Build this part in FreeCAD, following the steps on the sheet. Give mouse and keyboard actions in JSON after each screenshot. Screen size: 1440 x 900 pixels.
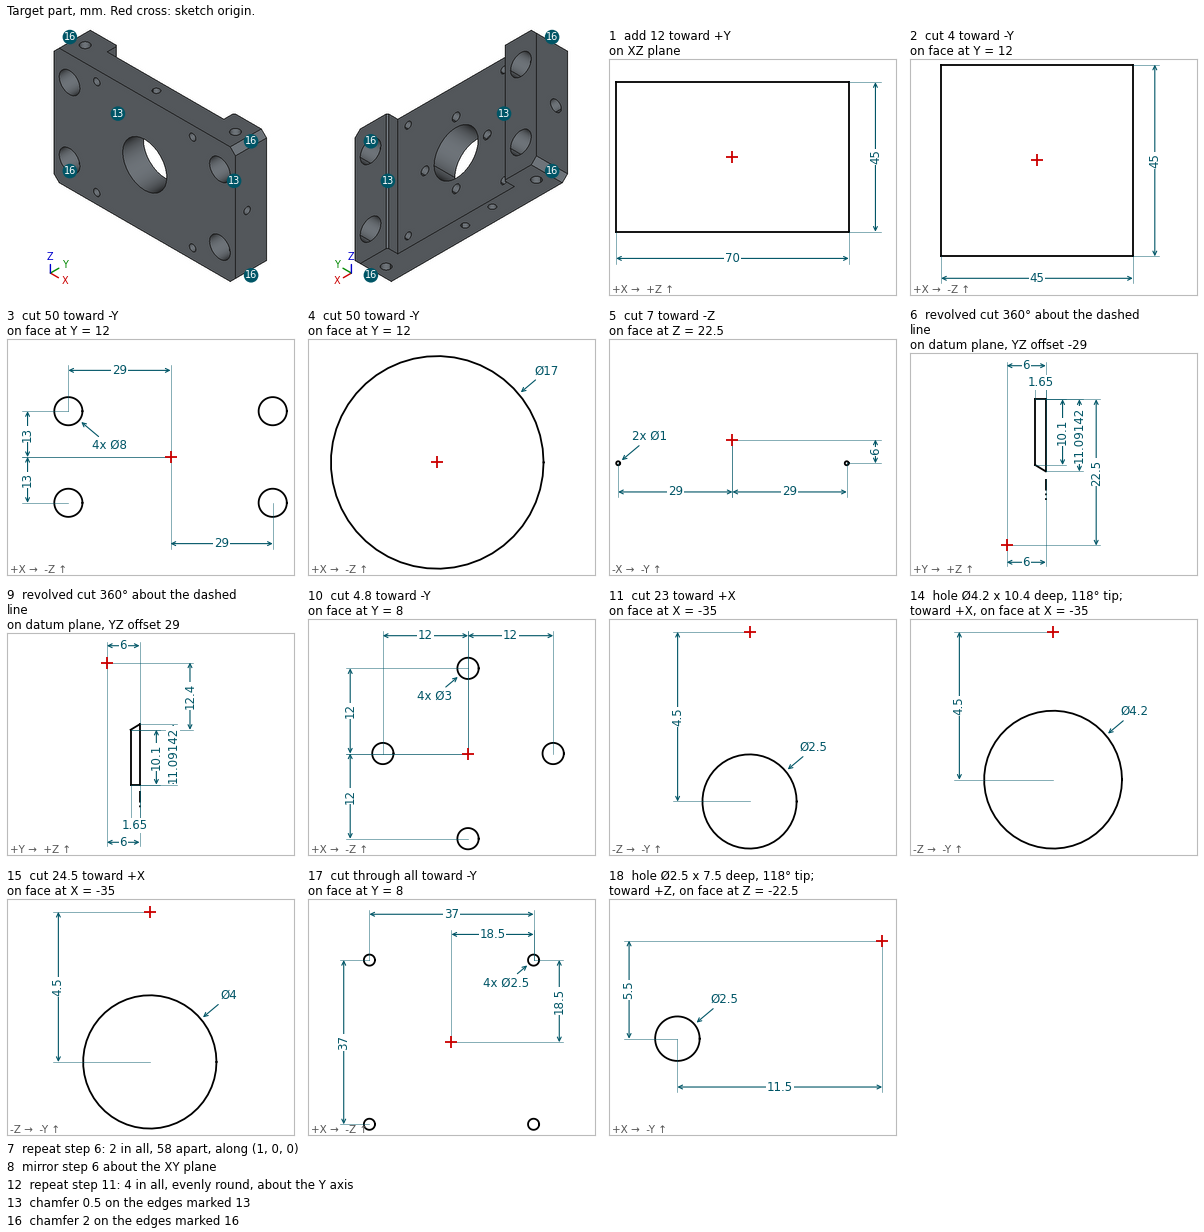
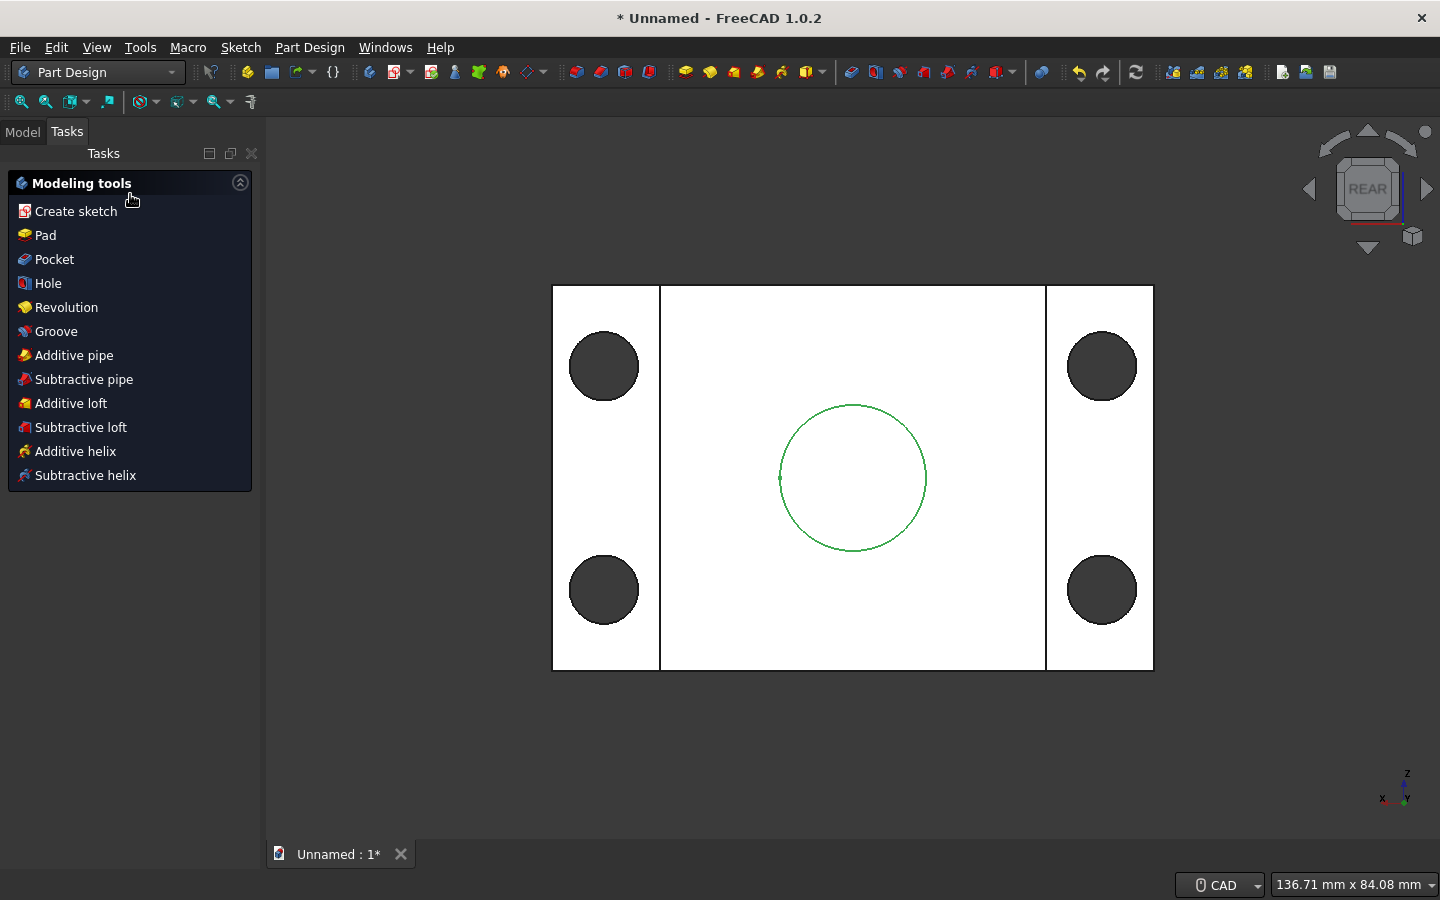
{"action": "left_click", "coordinate": [852, 72]}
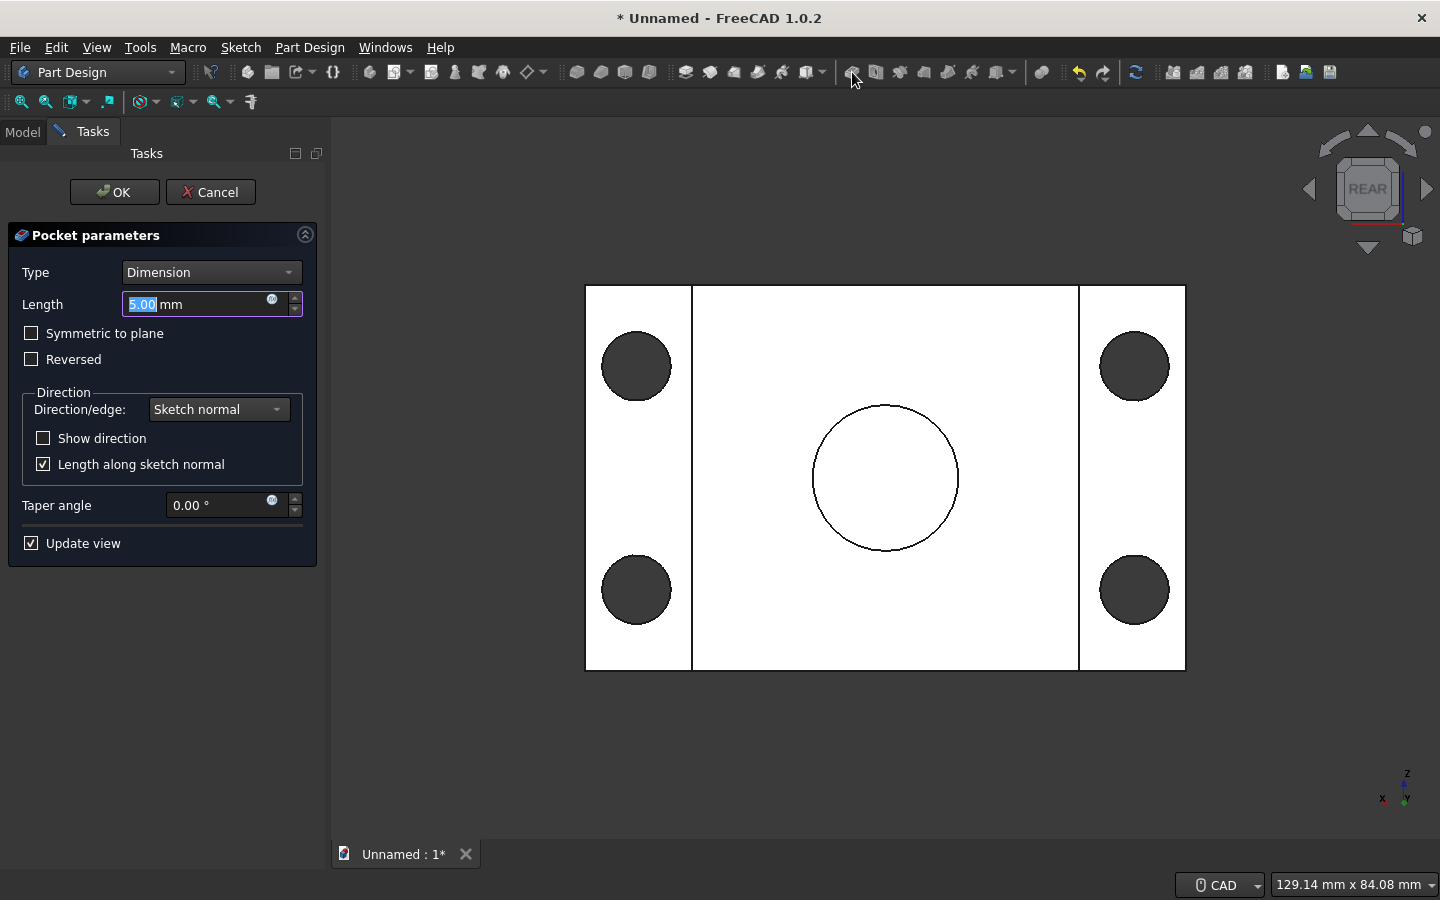
{"action": "type", "text": "50"}
{"action": "key", "text": "Tab"}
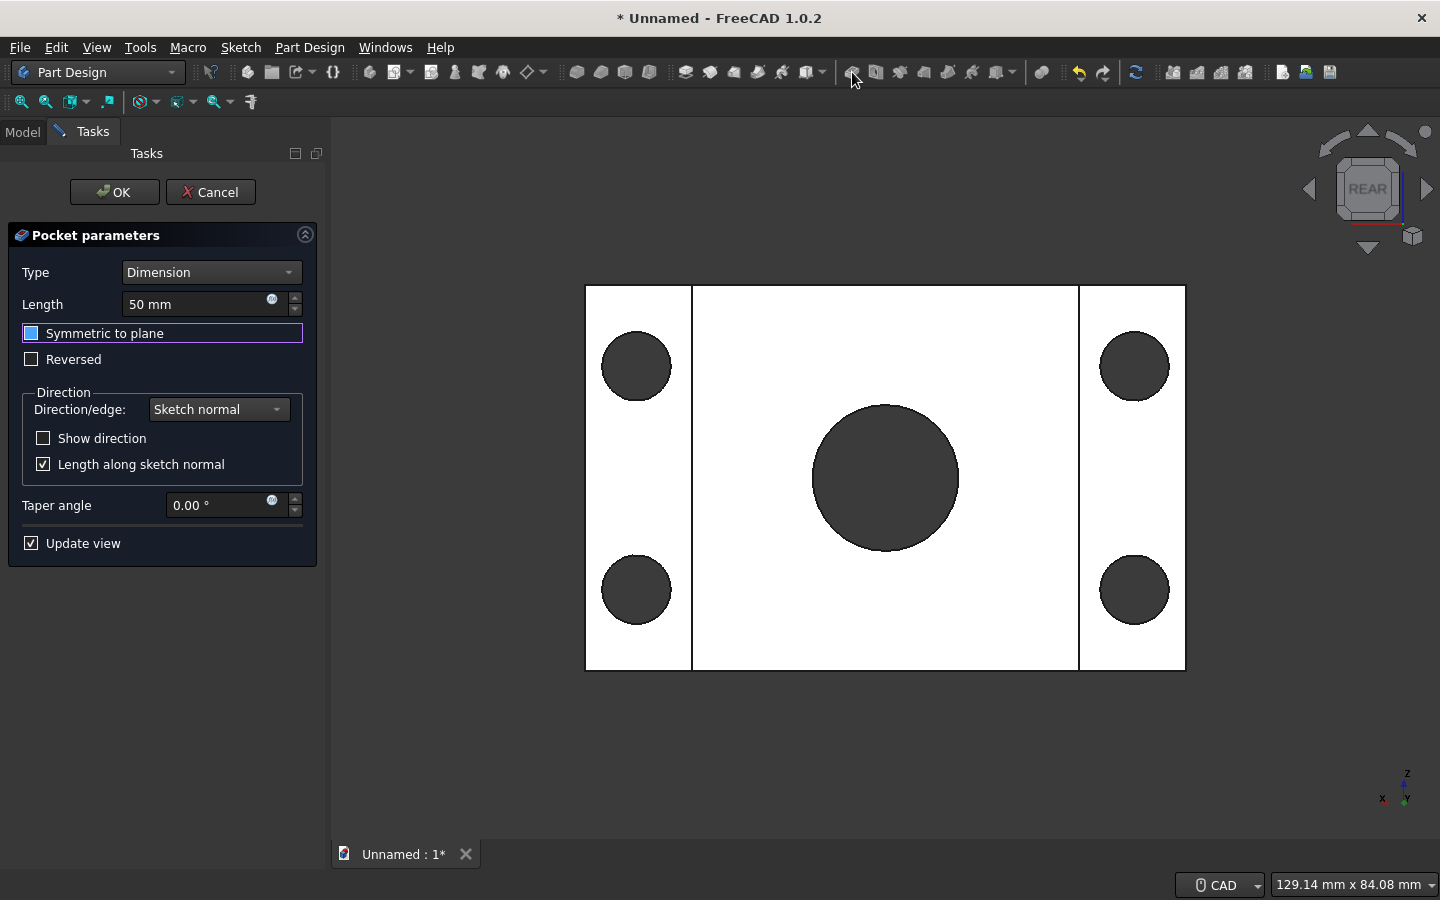
{"action": "left_click", "coordinate": [115, 192]}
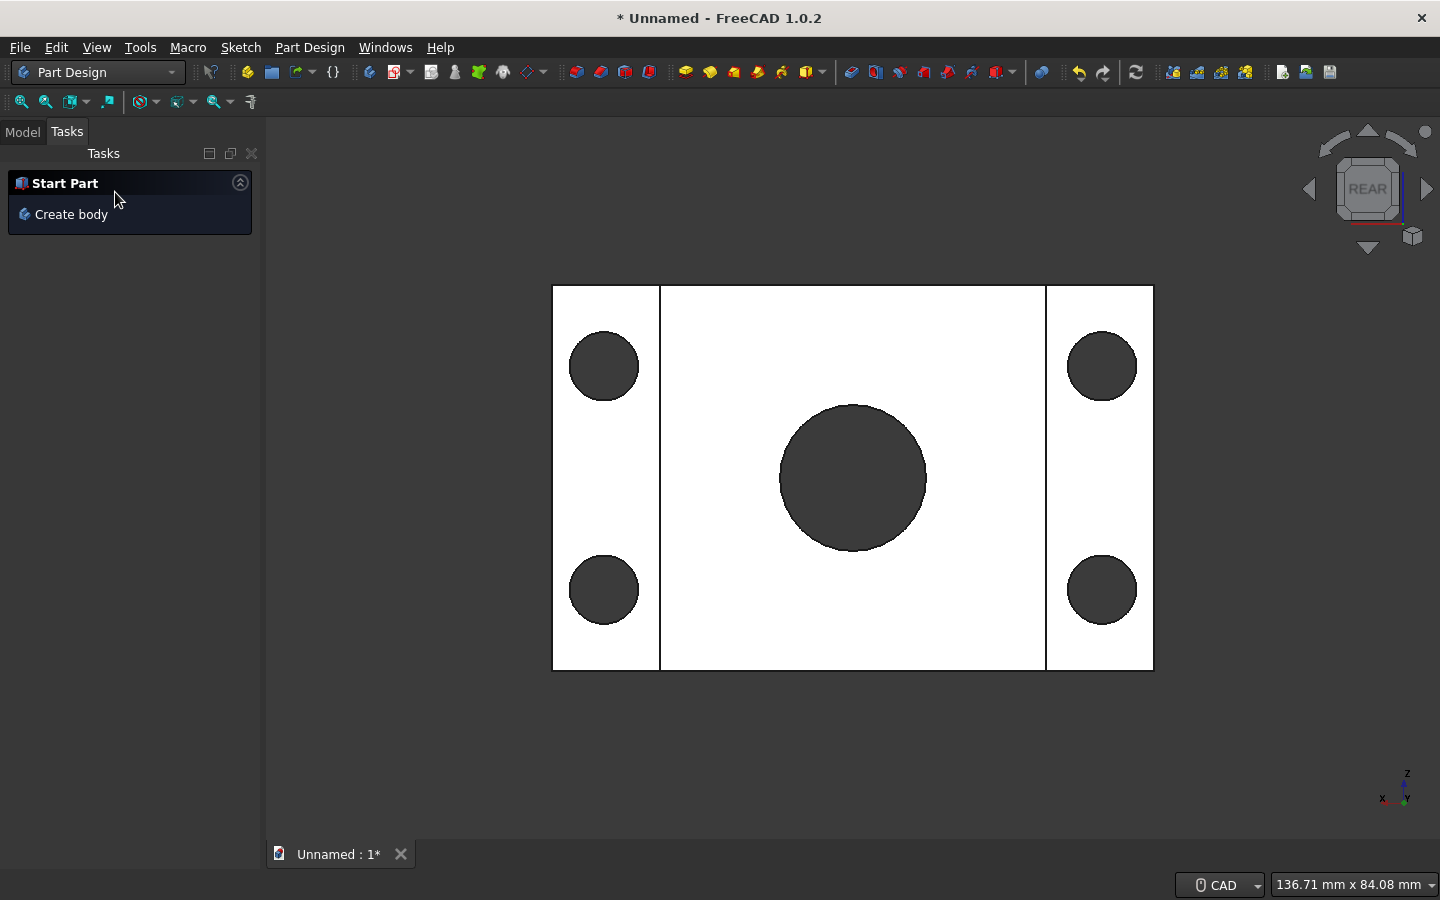
{"action": "key", "text": "0"}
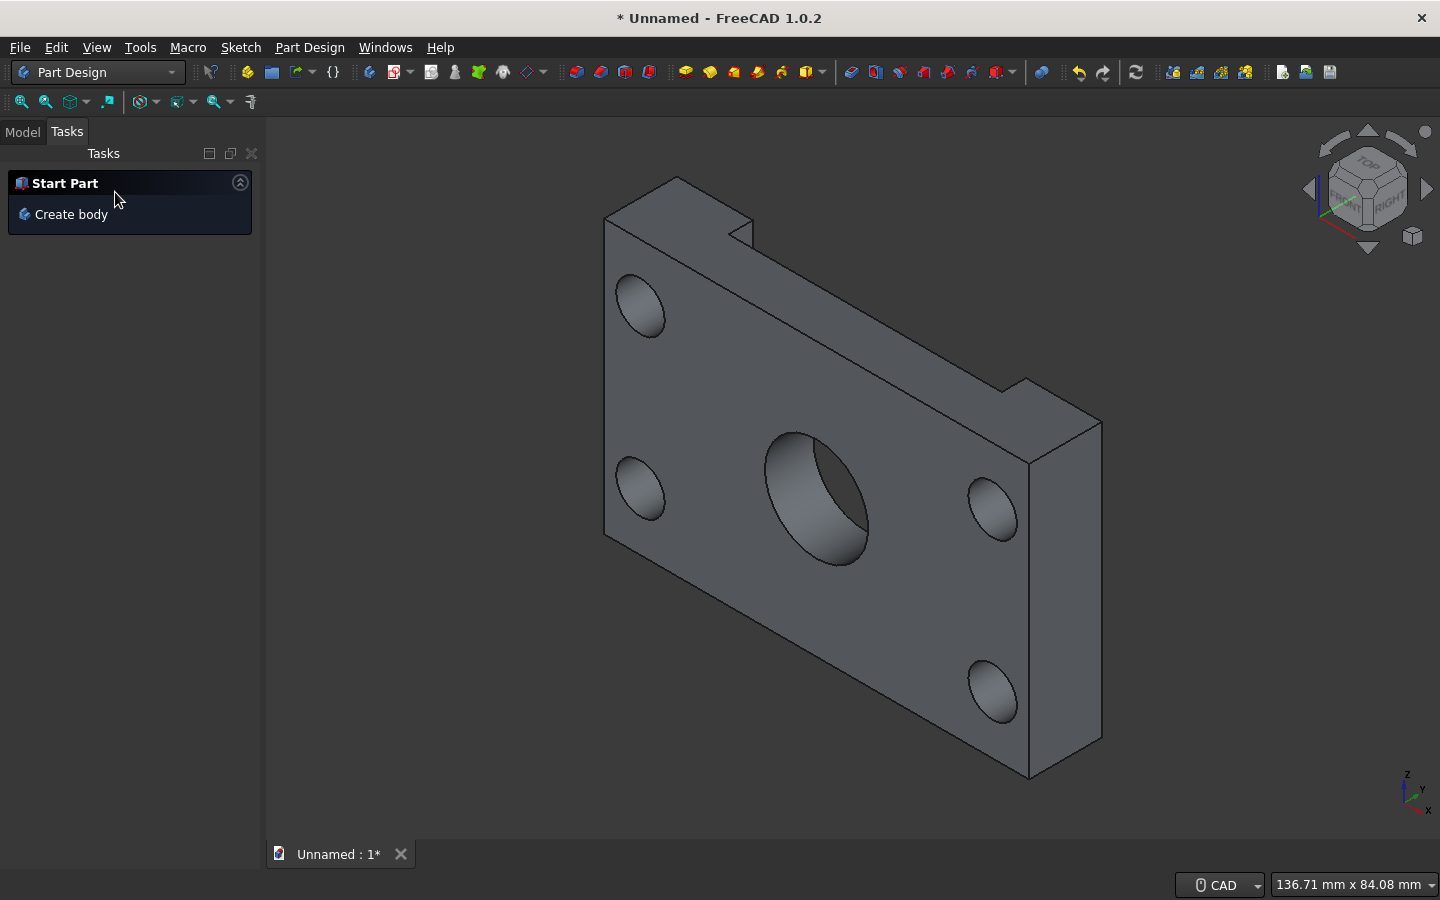
{"action": "left_click", "coordinate": [1035, 424]}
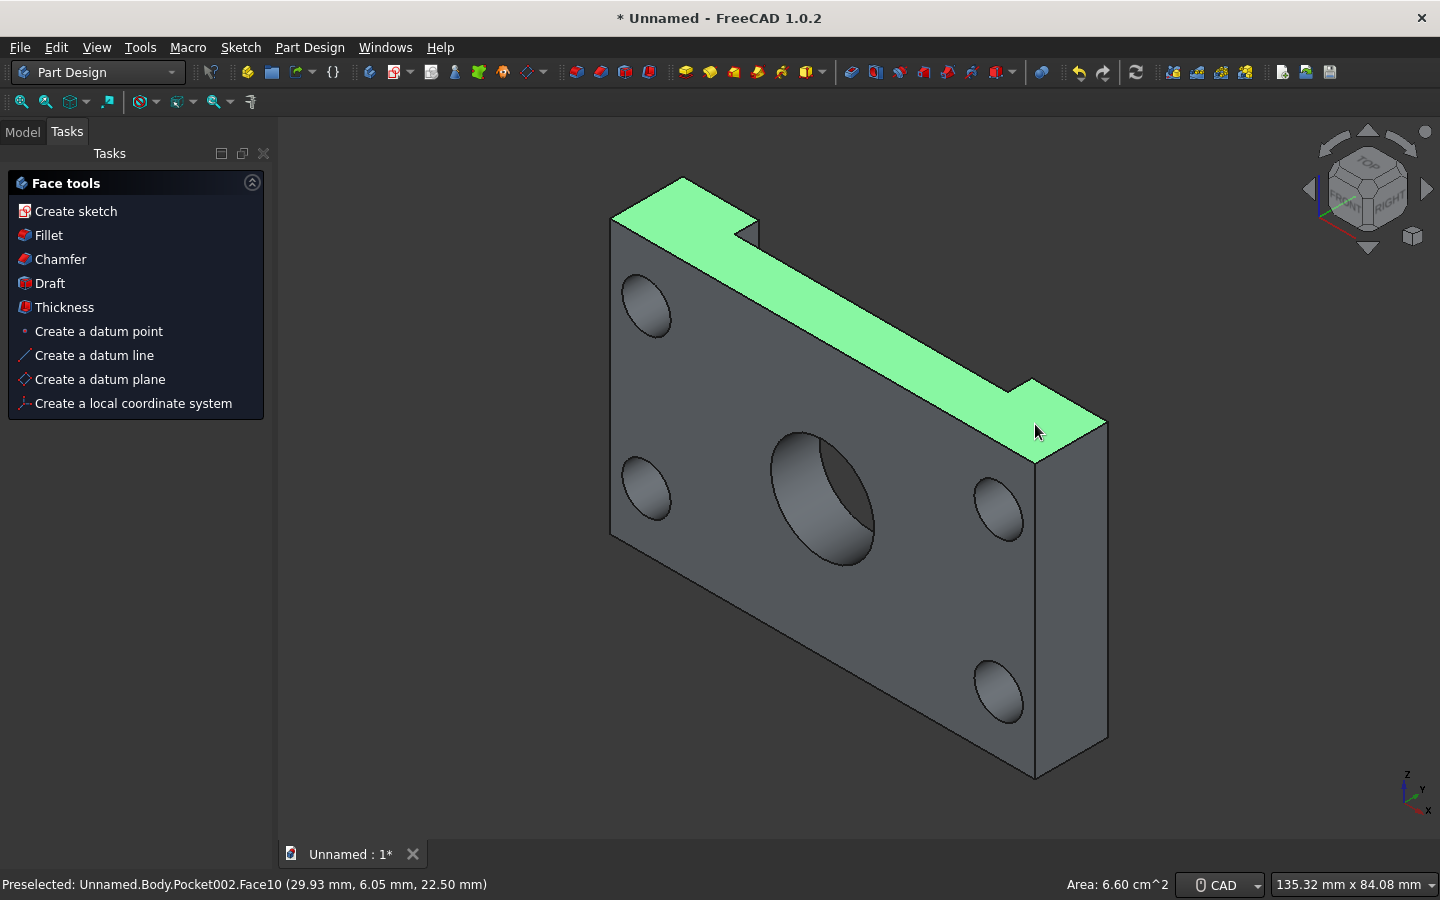
{"action": "left_click", "coordinate": [394, 72]}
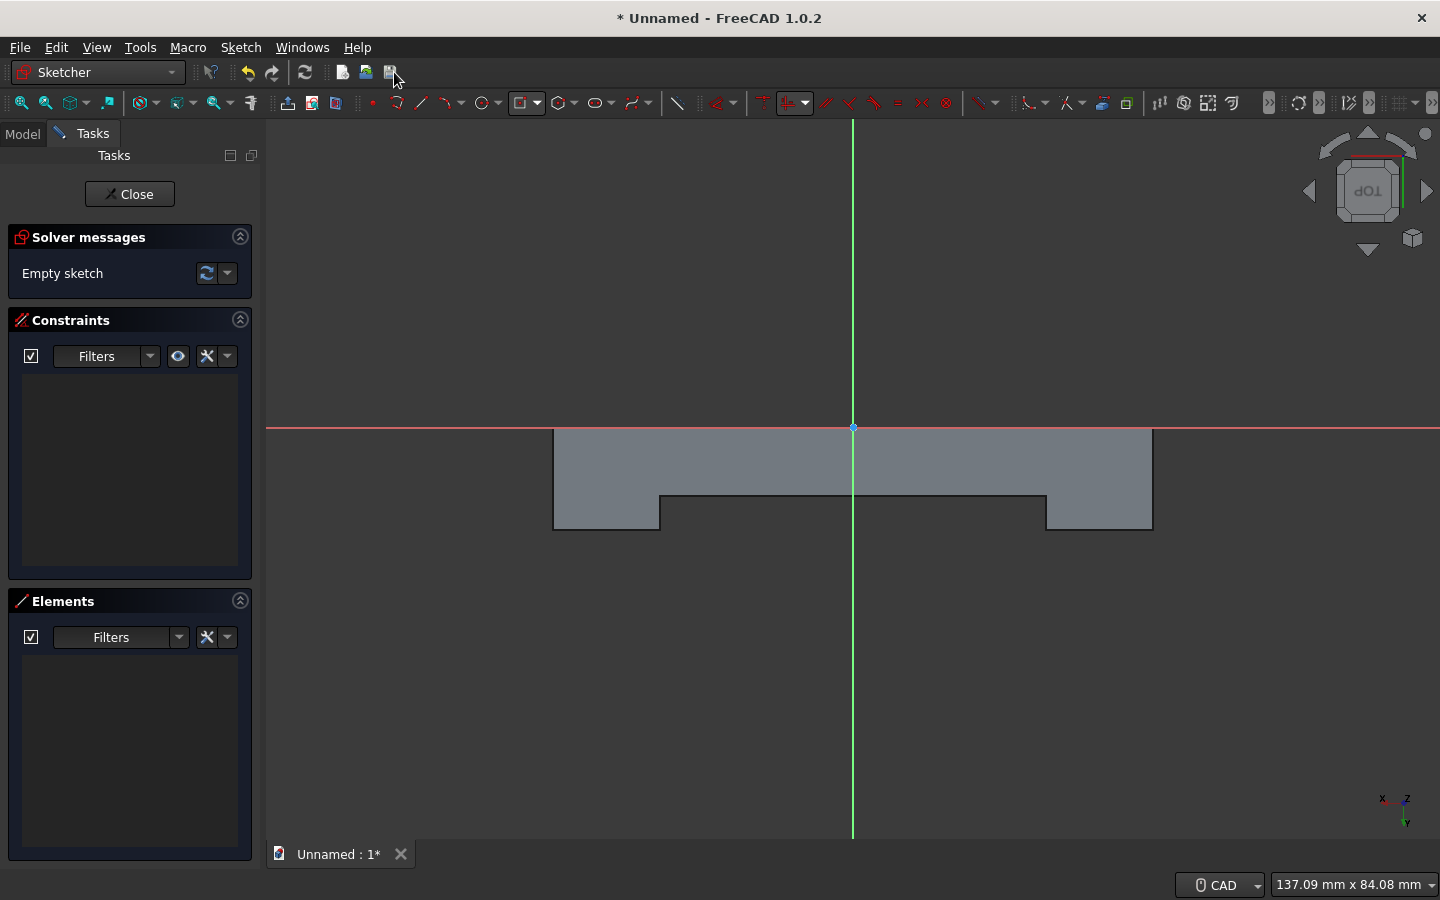
{"action": "scroll", "coordinate": [992, 408], "scroll_direction": "up", "scroll_amount": 2}